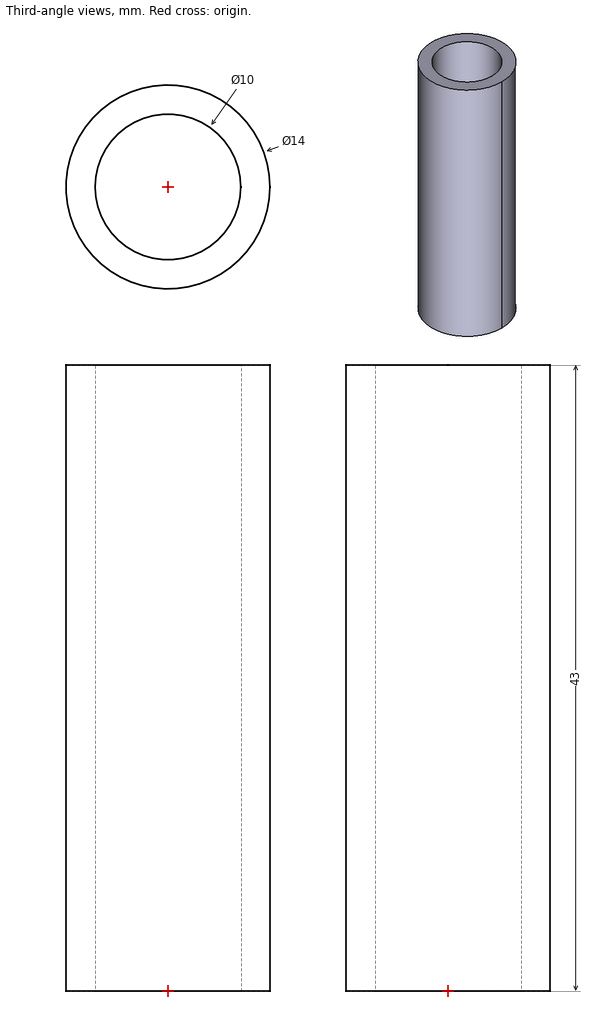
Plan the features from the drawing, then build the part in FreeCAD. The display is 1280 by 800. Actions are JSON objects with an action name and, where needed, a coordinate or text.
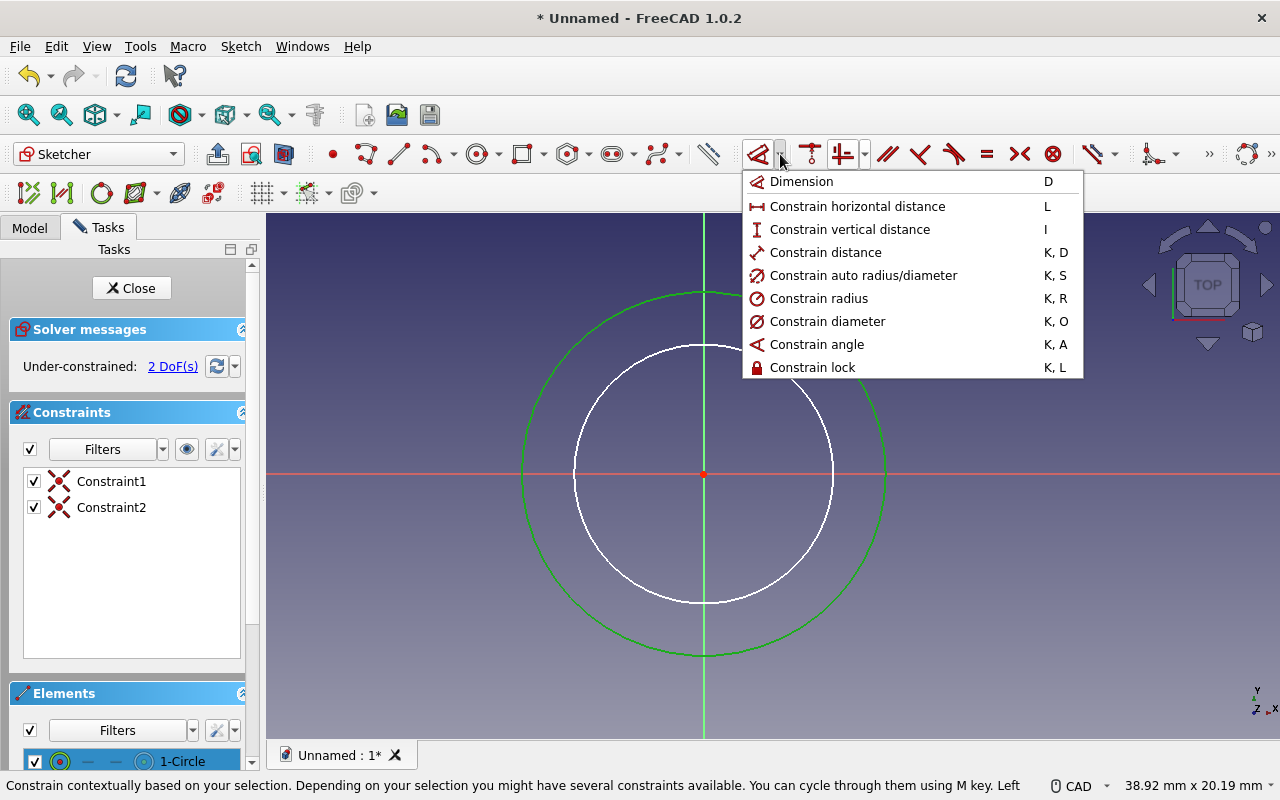
{"action": "left_click", "coordinate": [913, 322]}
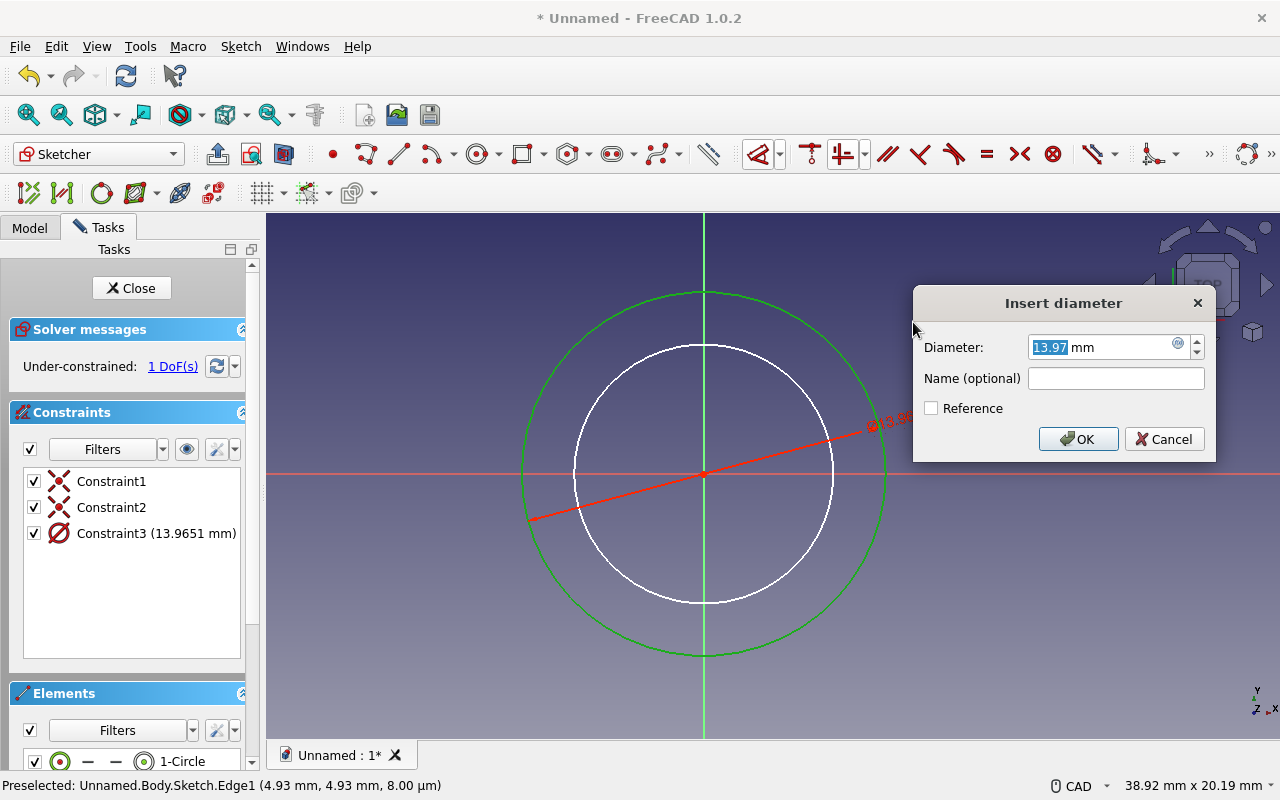
{"action": "type", "text": "14"}
{"action": "key", "text": "Return"}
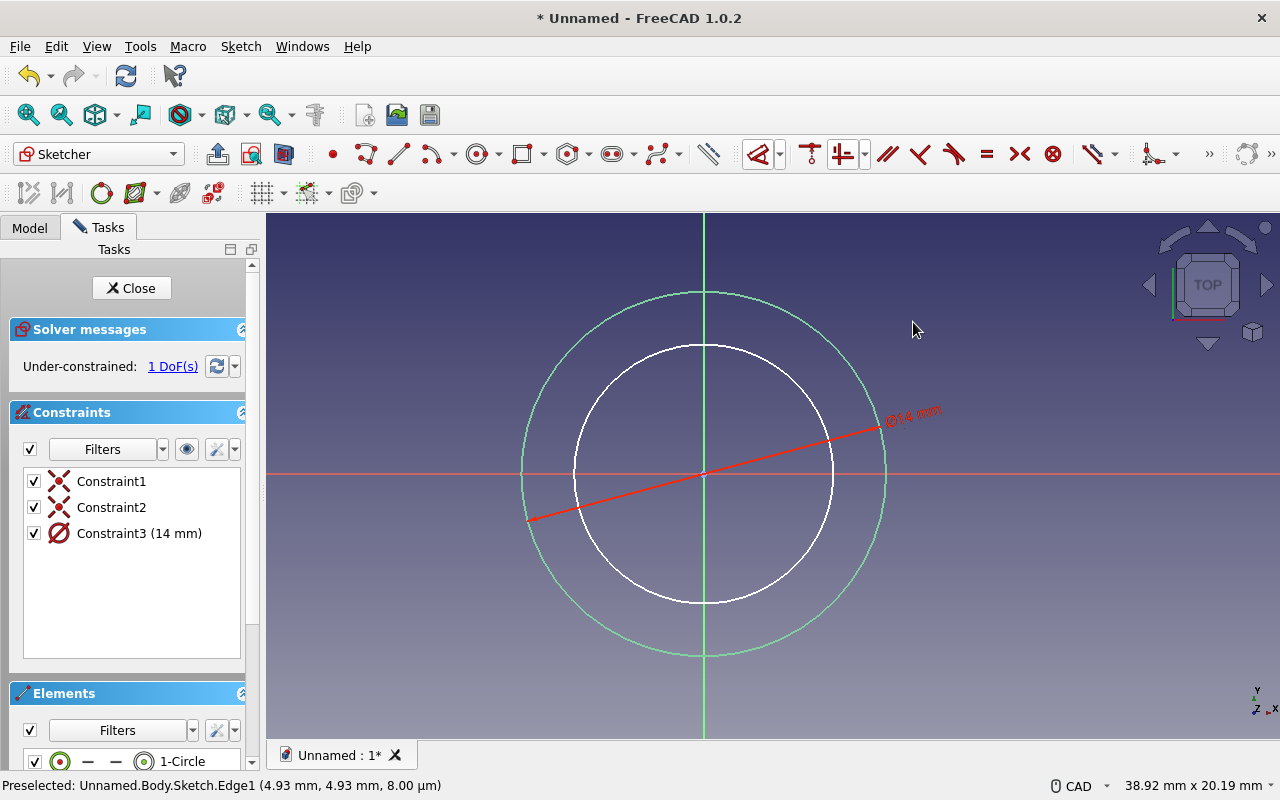
{"action": "left_click", "coordinate": [795, 382]}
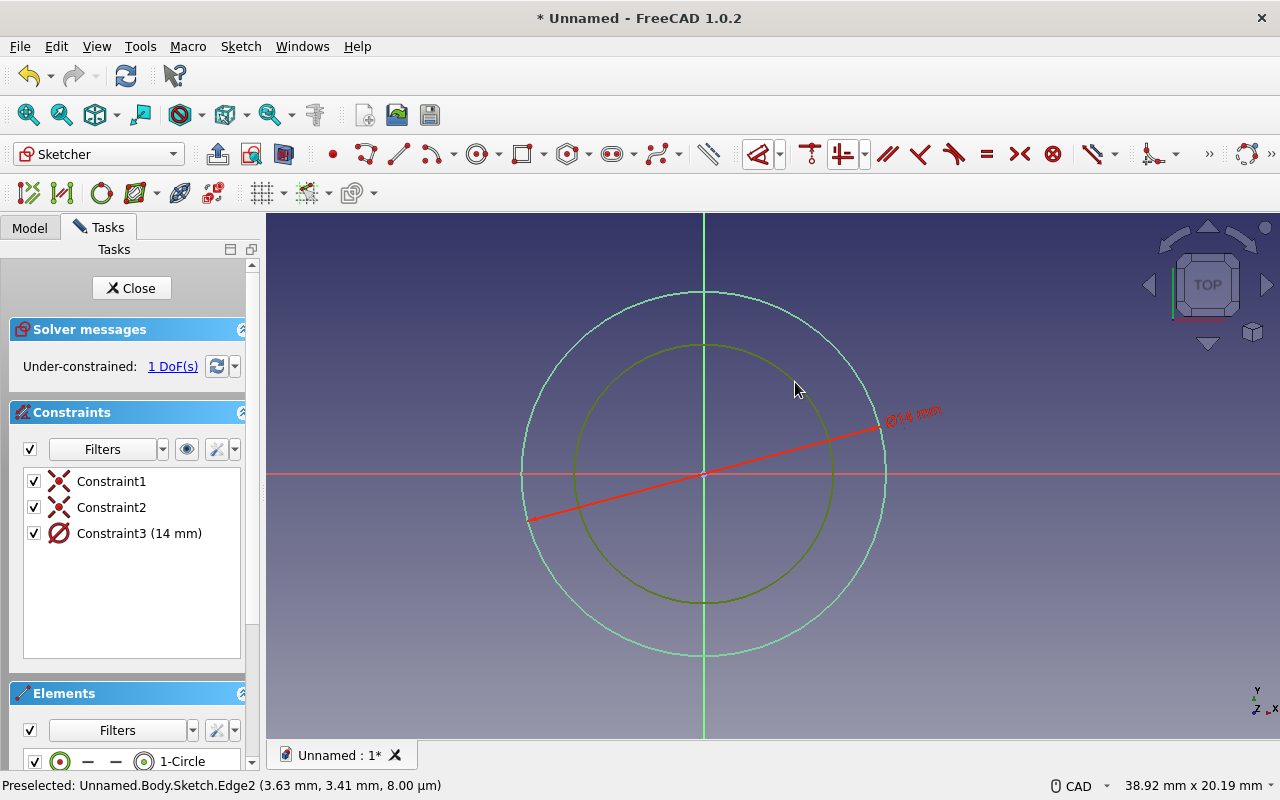
{"action": "left_click", "coordinate": [780, 154]}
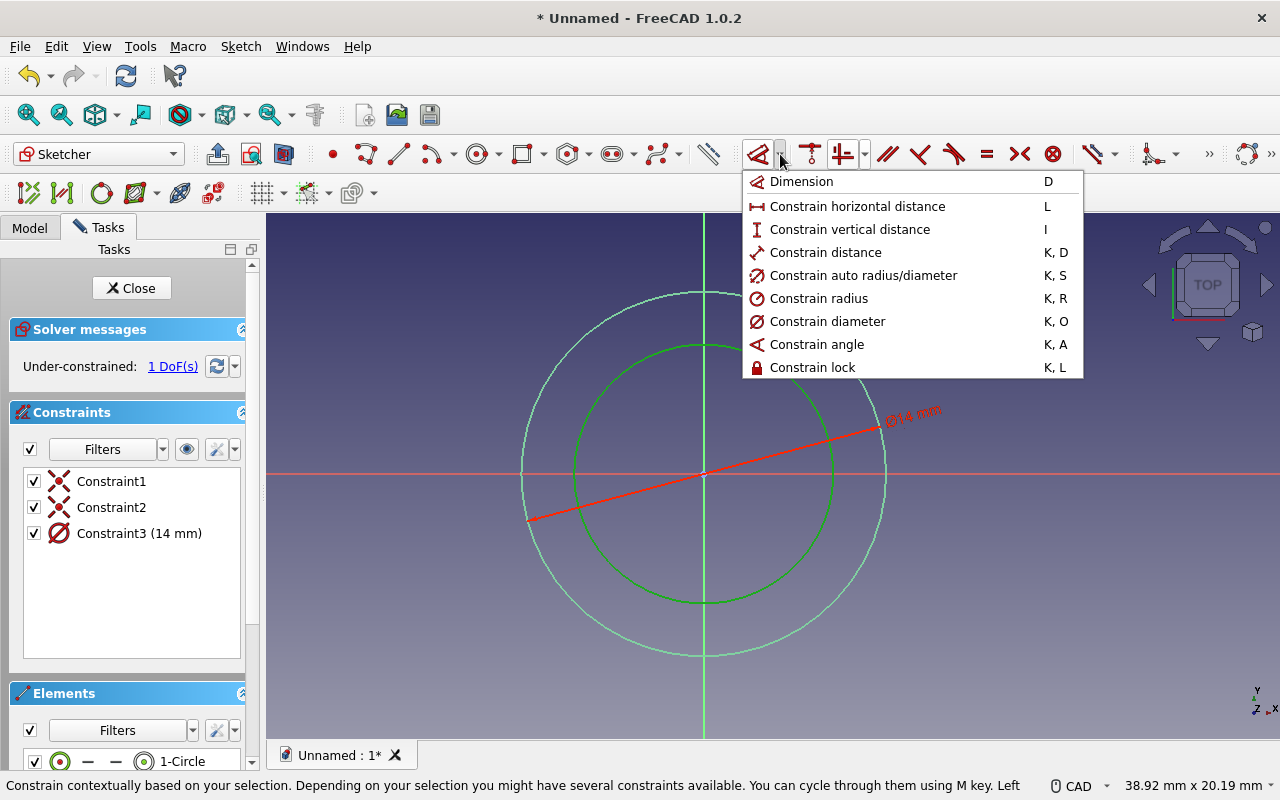
{"action": "left_click", "coordinate": [913, 322]}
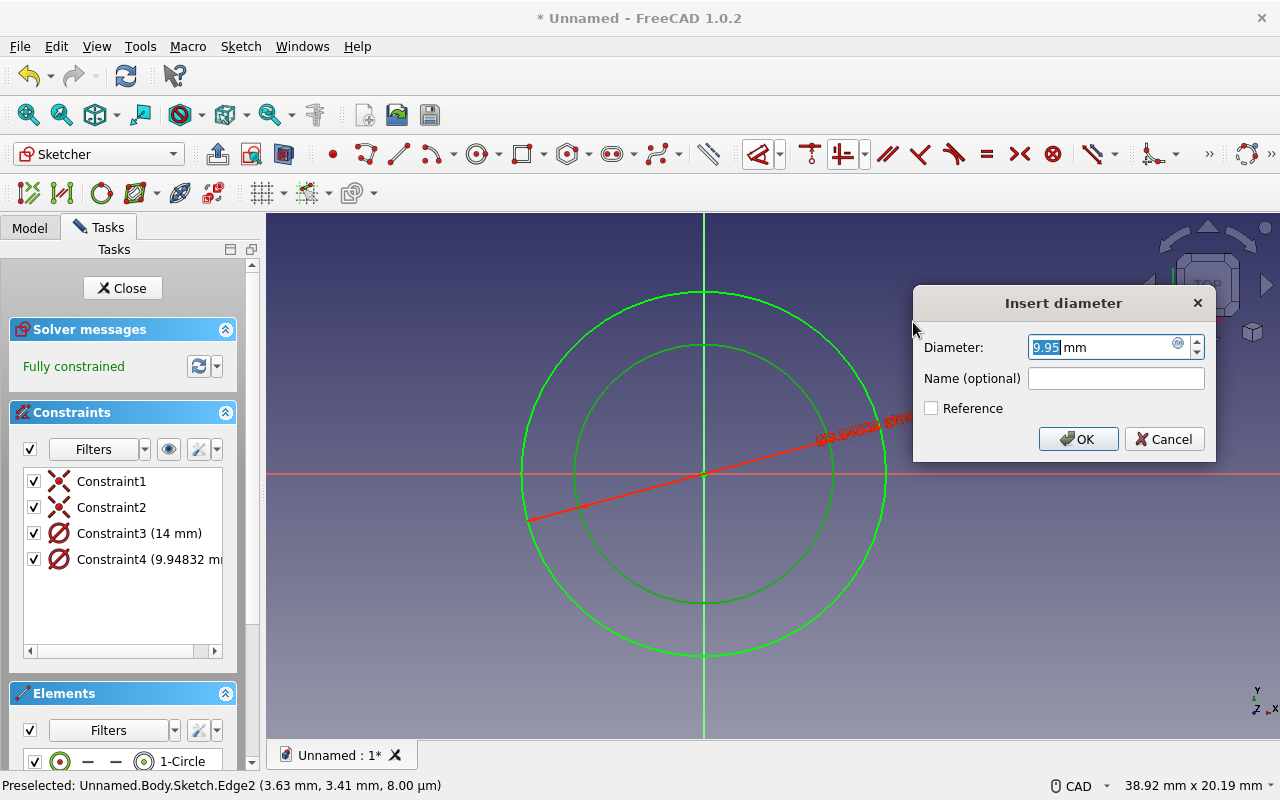
{"action": "type", "text": "10"}
{"action": "key", "text": "Return"}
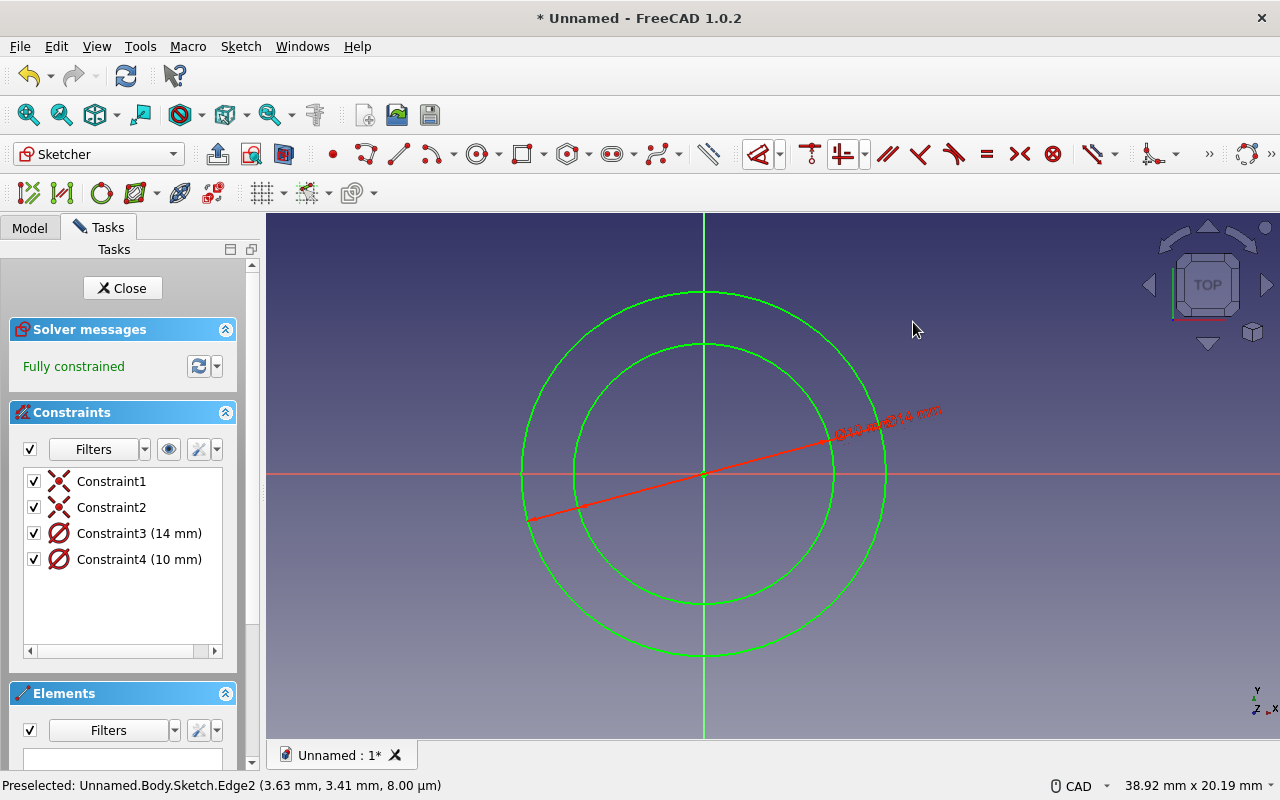
{"action": "left_click", "coordinate": [123, 288]}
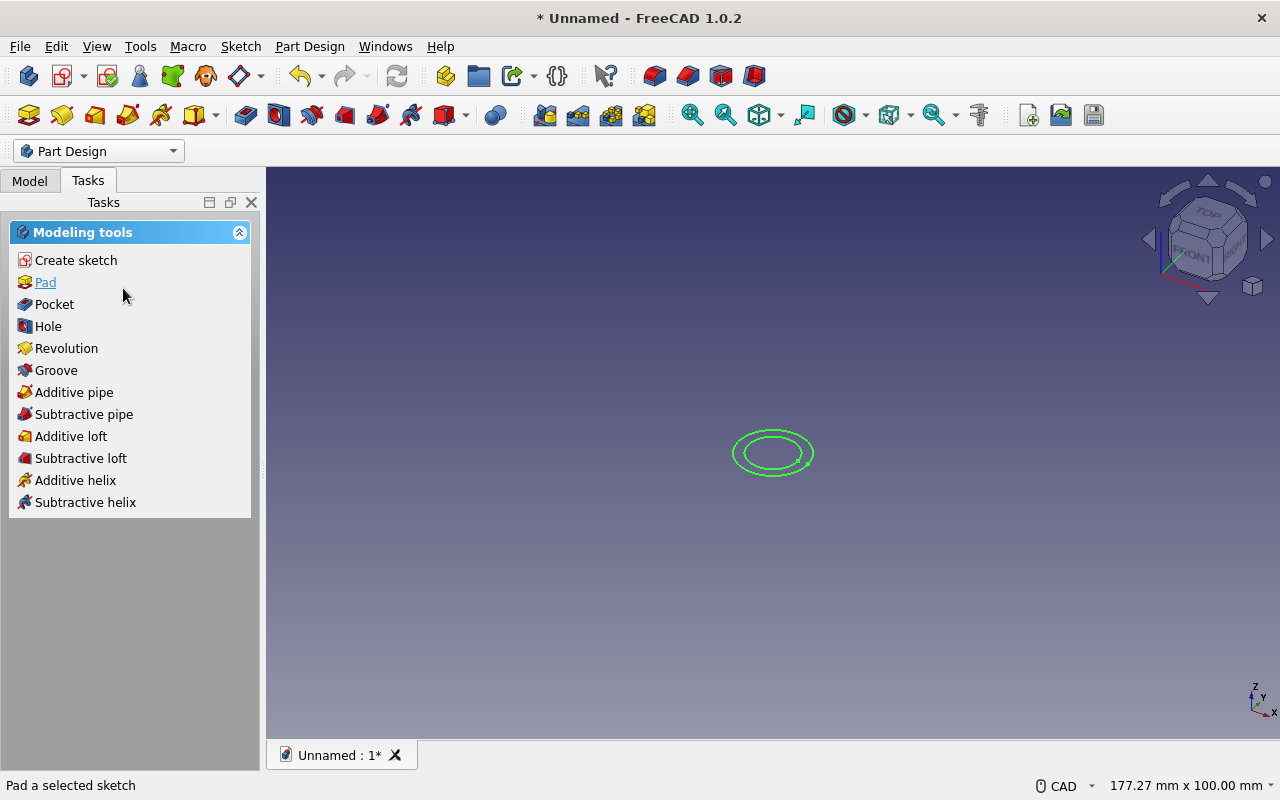
{"action": "left_click", "coordinate": [29, 116]}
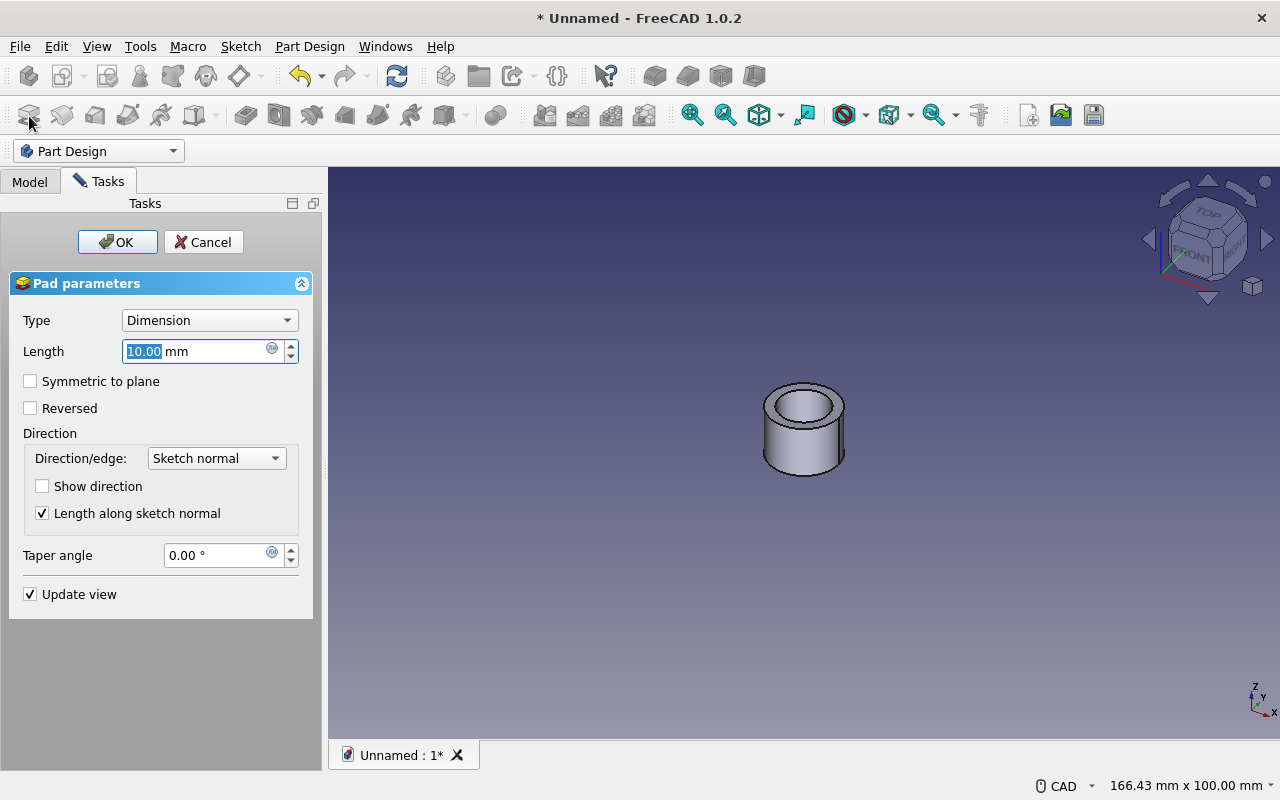
{"action": "type", "text": "43"}
{"action": "key", "text": "Tab"}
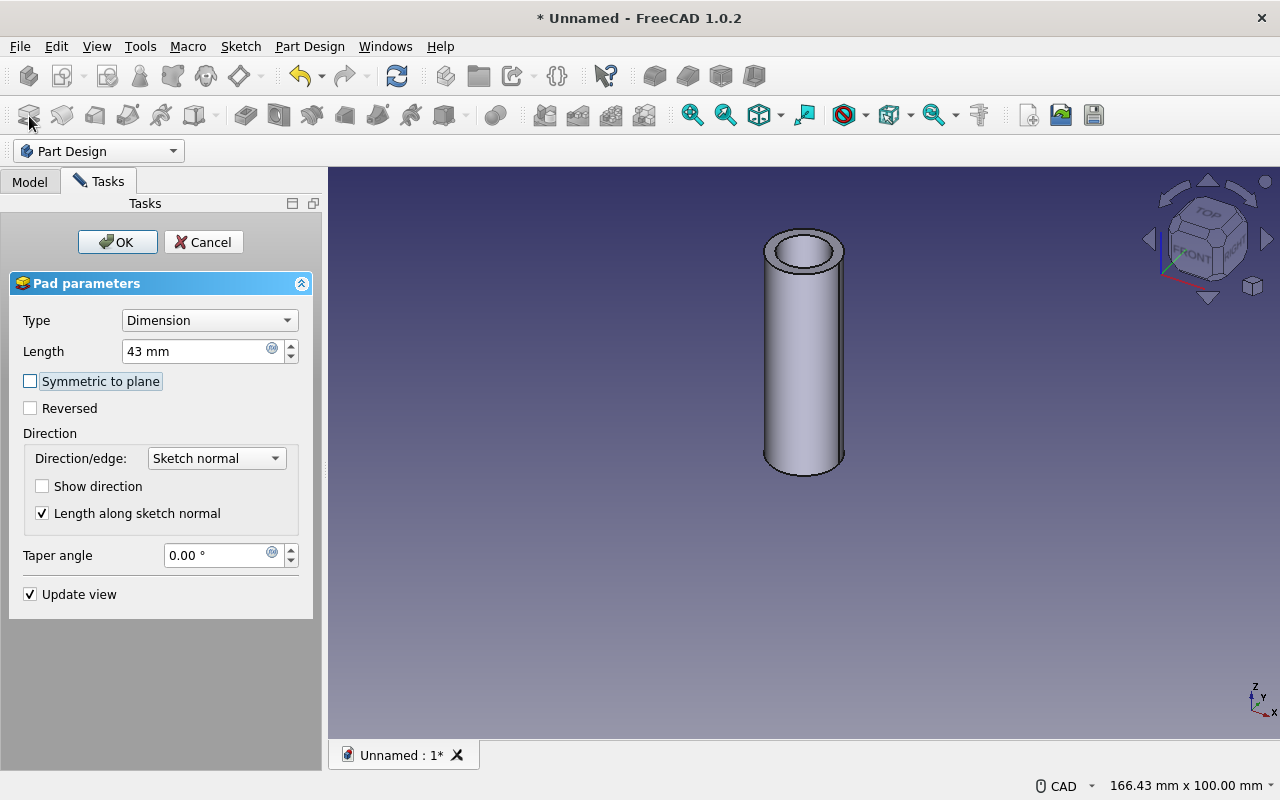
{"action": "left_click", "coordinate": [118, 242]}